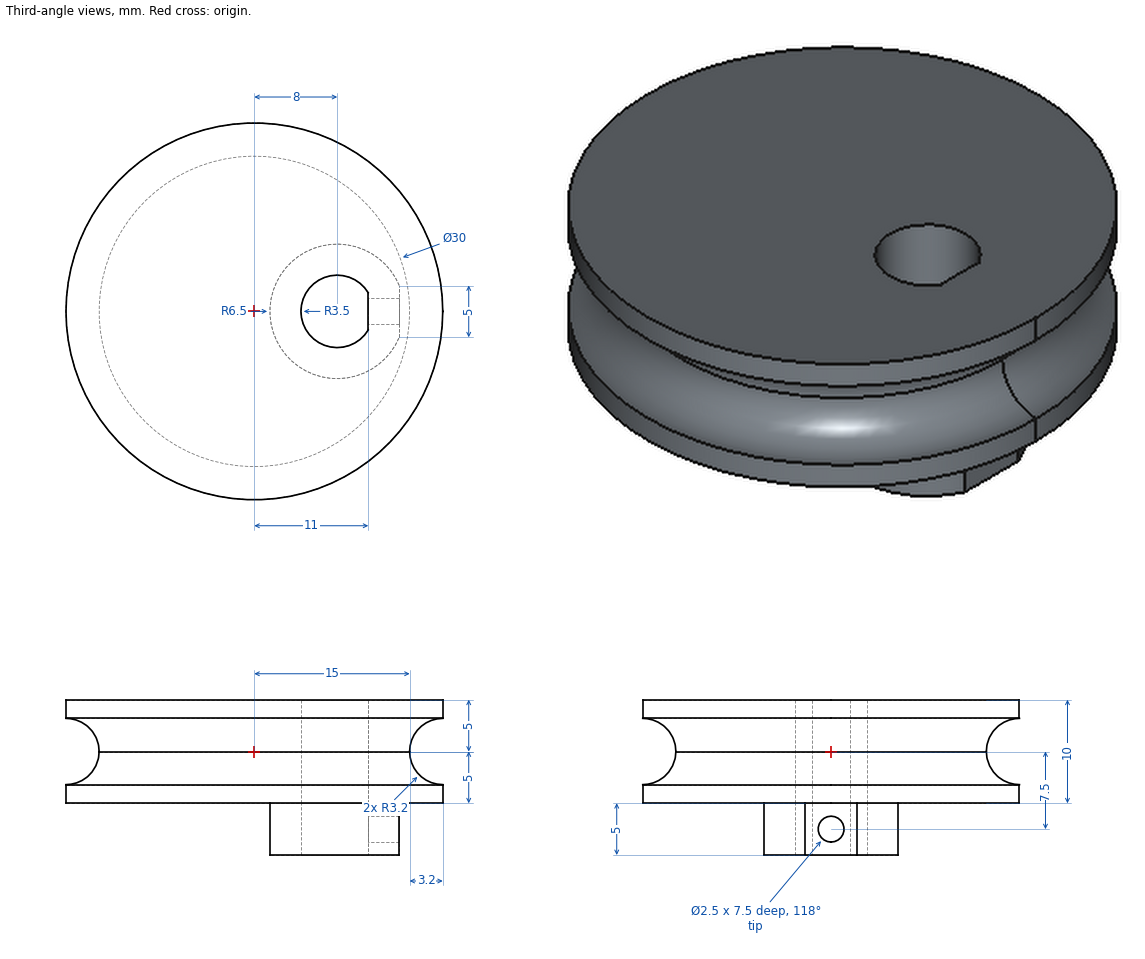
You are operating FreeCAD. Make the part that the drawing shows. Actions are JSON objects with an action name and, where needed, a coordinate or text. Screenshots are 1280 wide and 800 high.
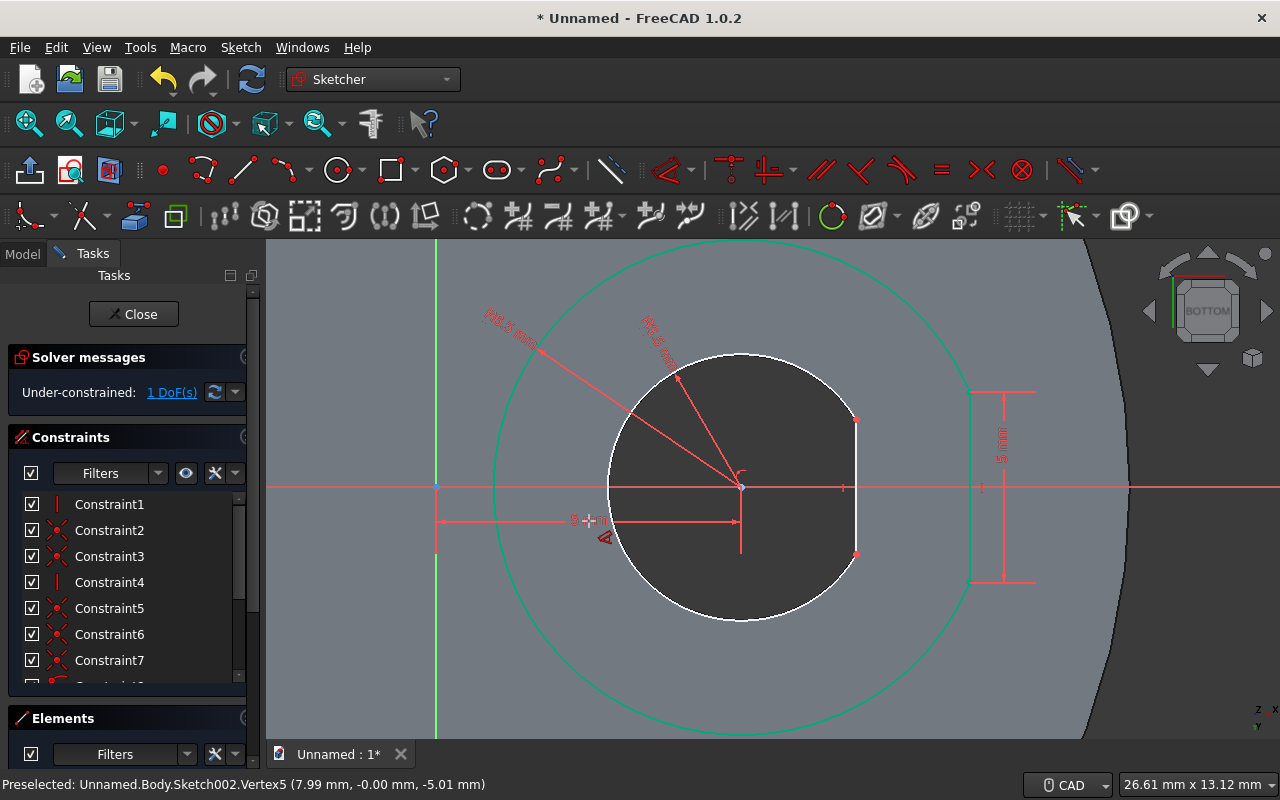
{"action": "left_click", "coordinate": [856, 555]}
{"action": "left_click", "coordinate": [550, 589]}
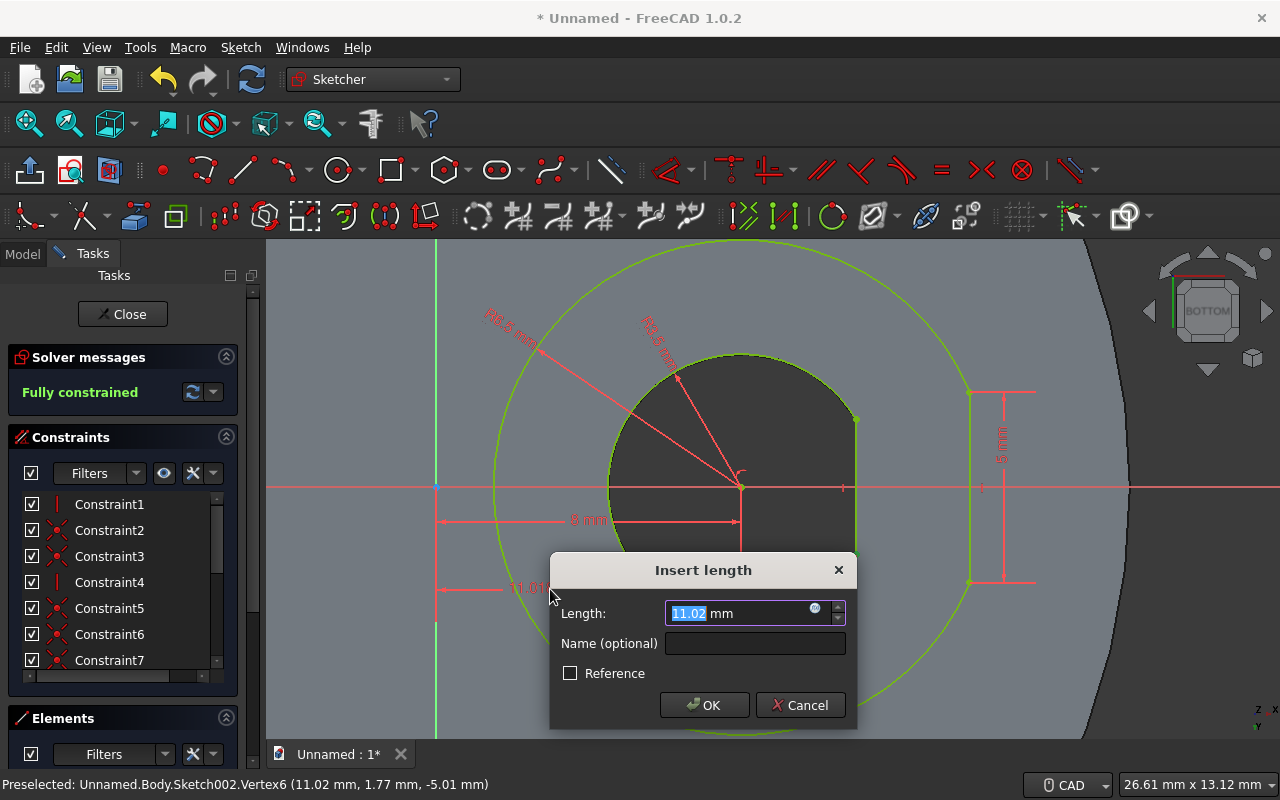
{"action": "type", "text": "11"}
{"action": "key", "text": "Return"}
{"action": "key", "text": "Escape"}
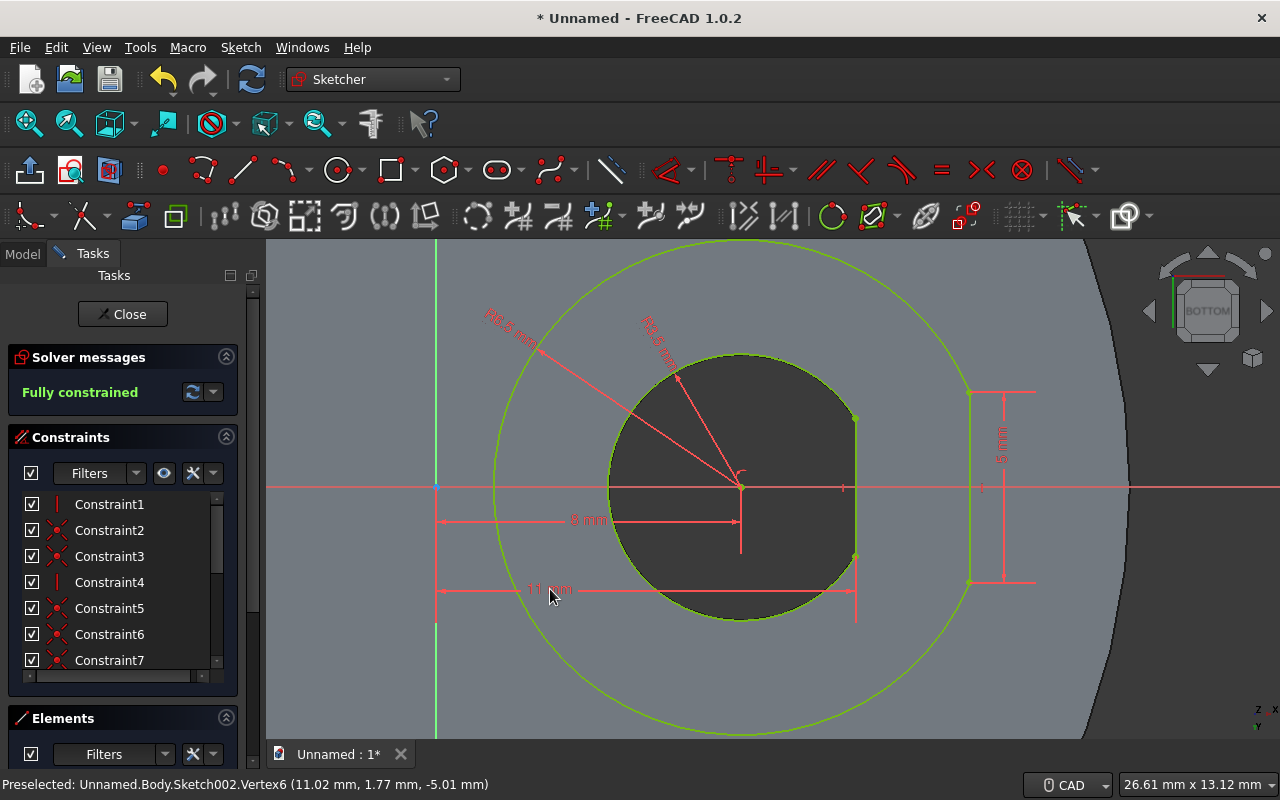
{"action": "left_click", "coordinate": [123, 314]}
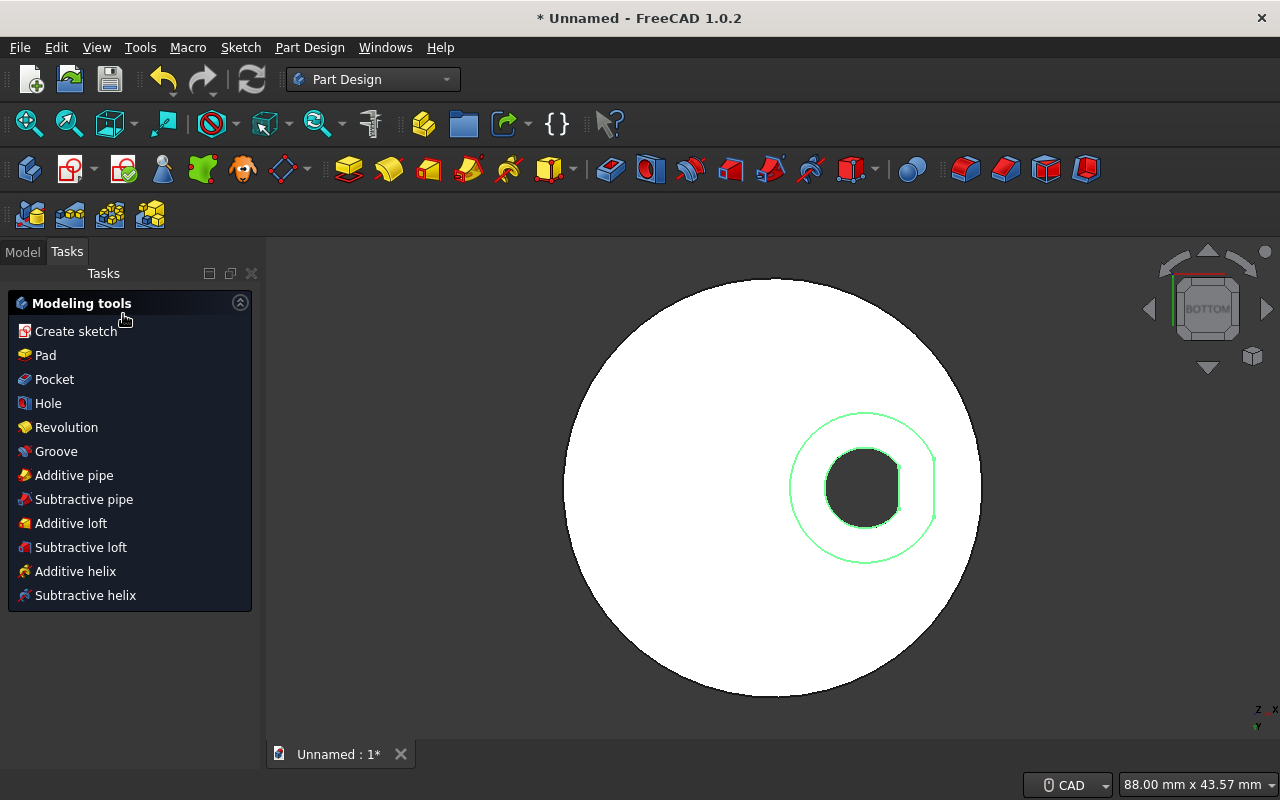
{"action": "left_click", "coordinate": [350, 170]}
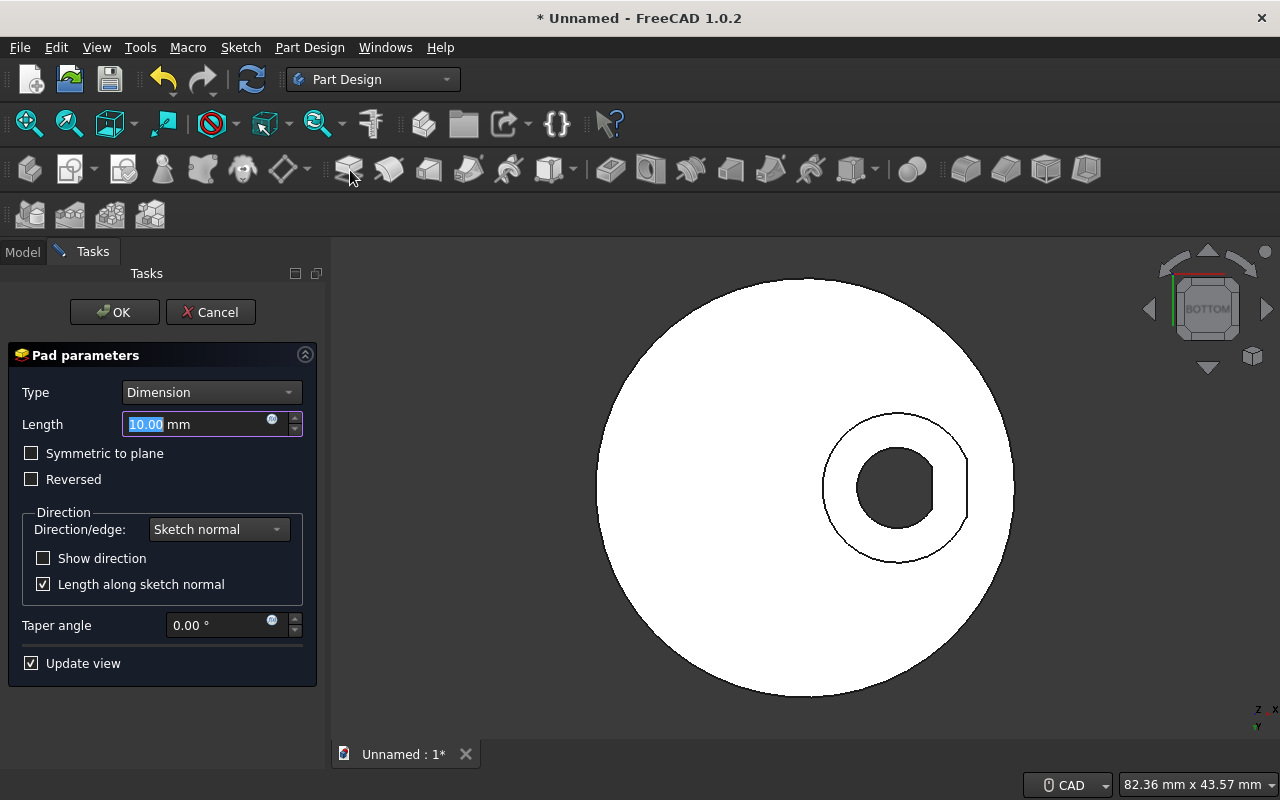
{"action": "type", "text": "5"}
{"action": "key", "text": "Tab"}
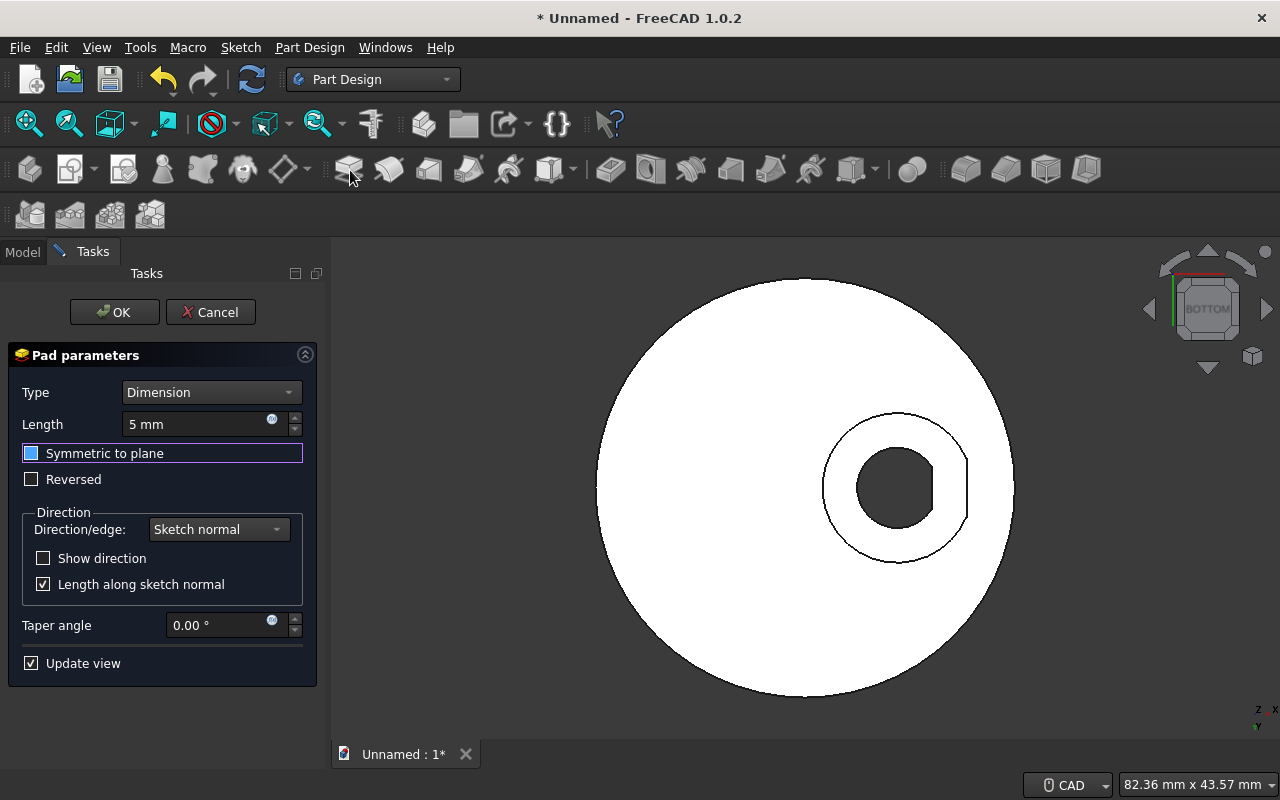
{"action": "left_click", "coordinate": [115, 312]}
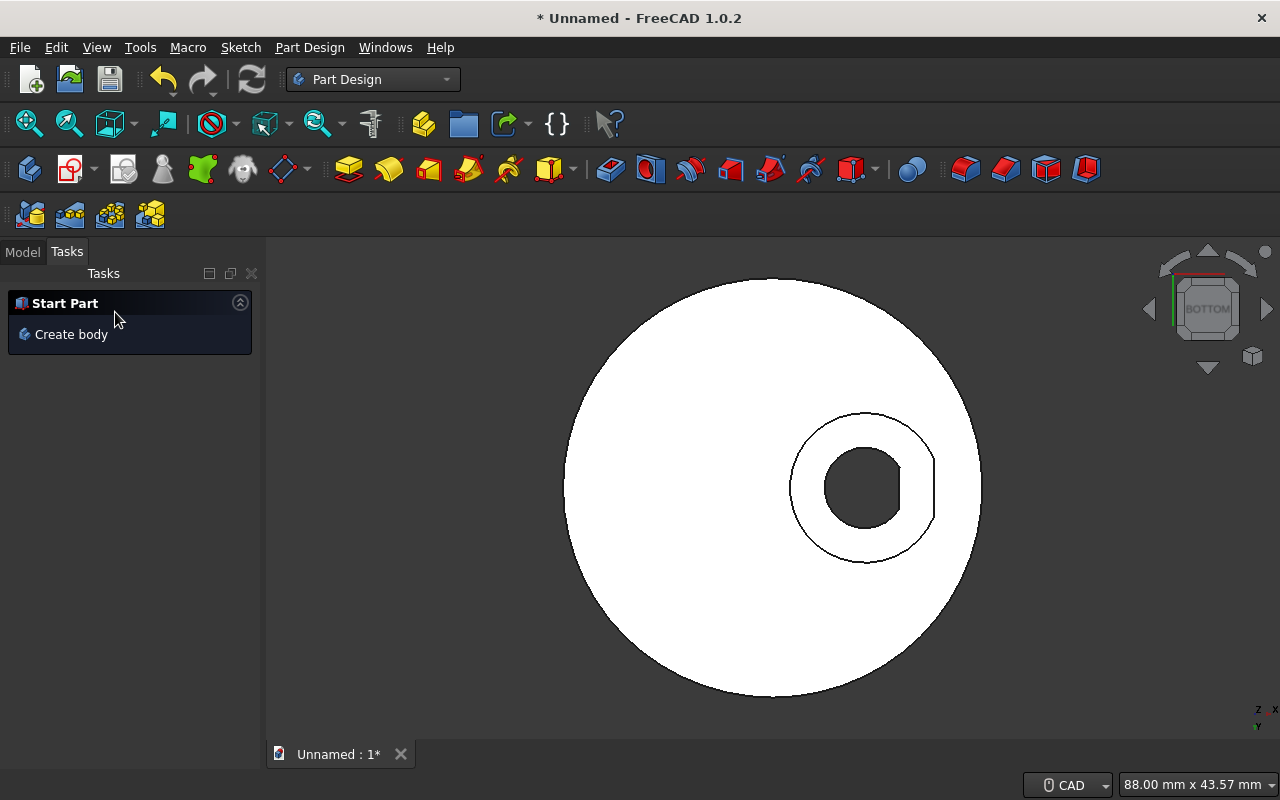
{"action": "key", "text": "0"}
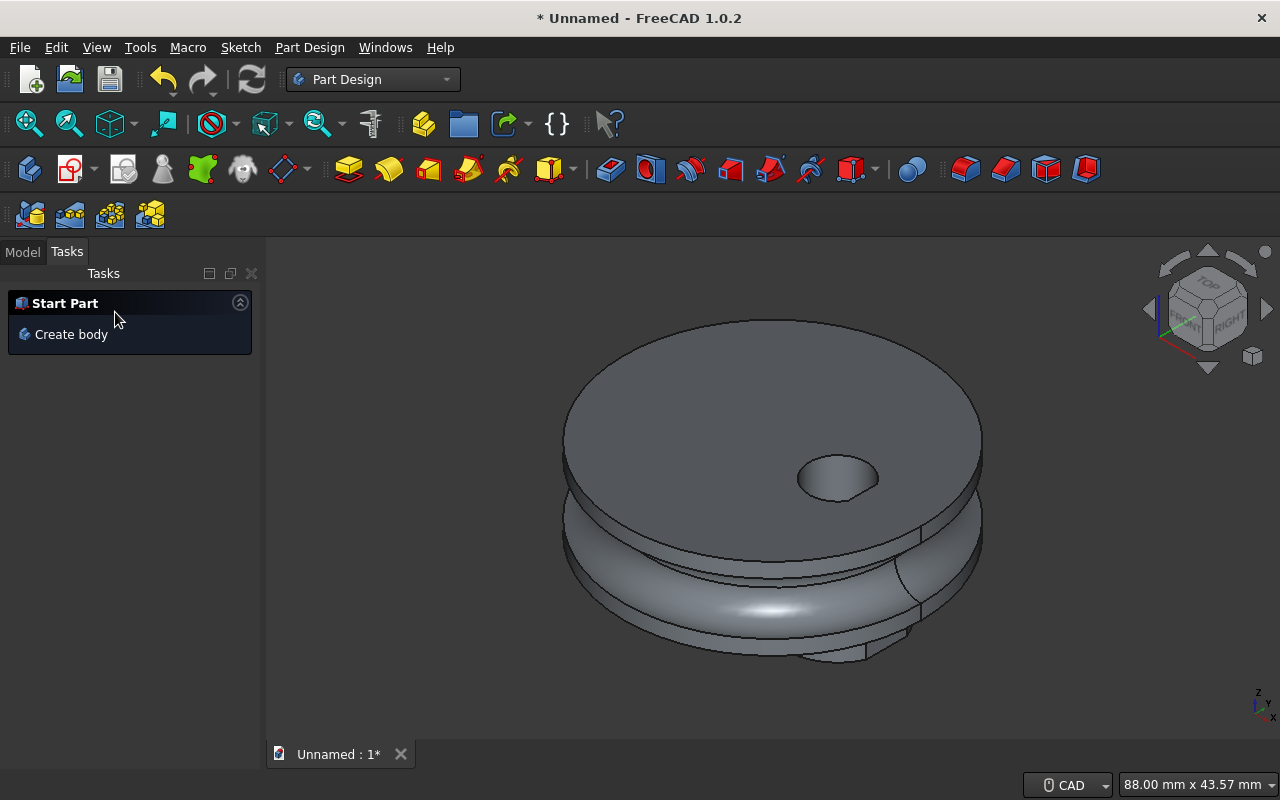
{"action": "left_click", "coordinate": [30, 124]}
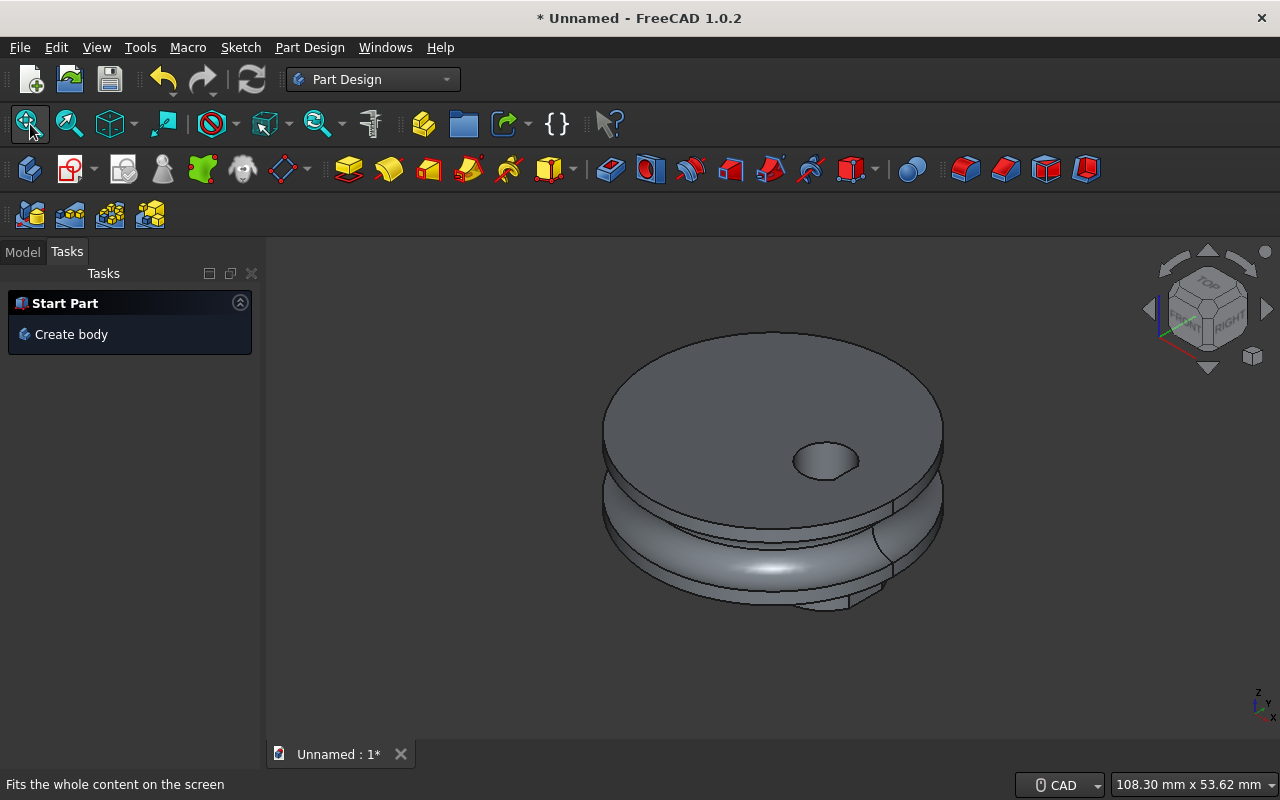
{"action": "key", "text": "3"}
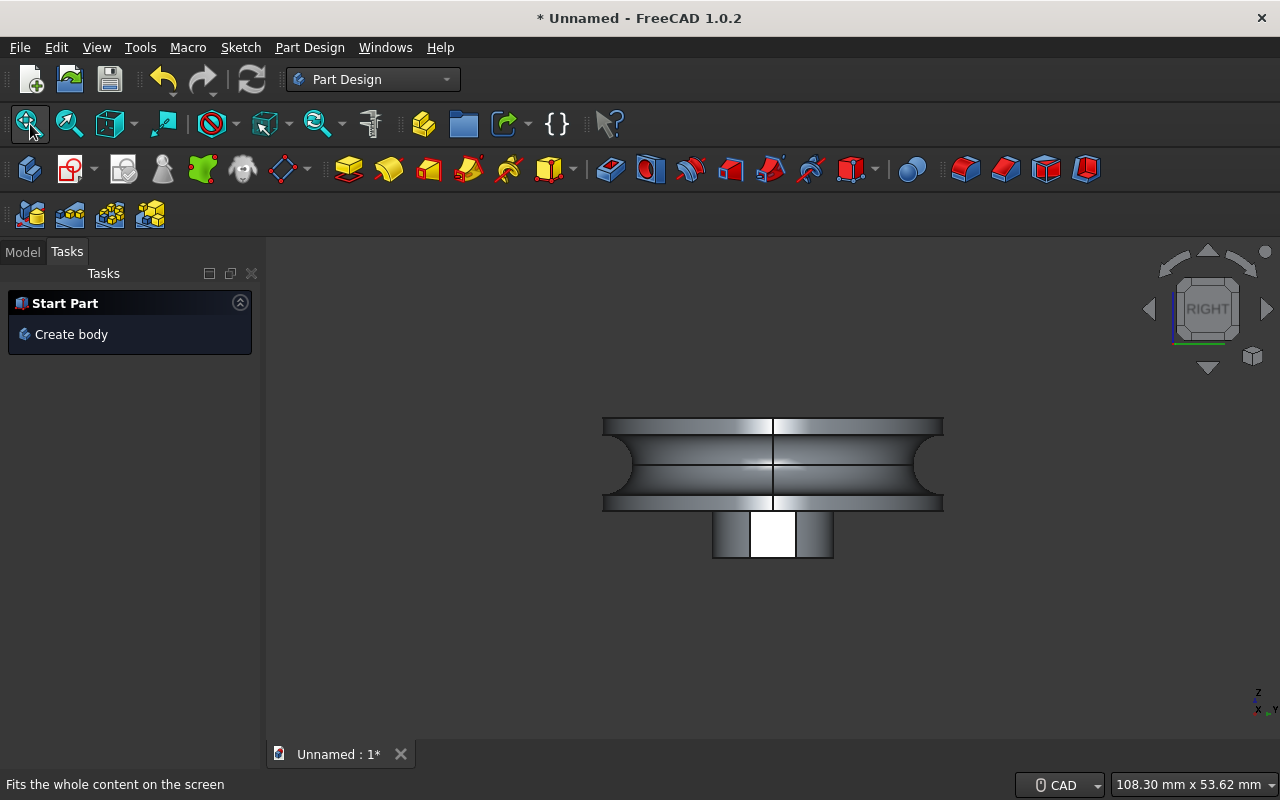
{"action": "left_click", "coordinate": [30, 124]}